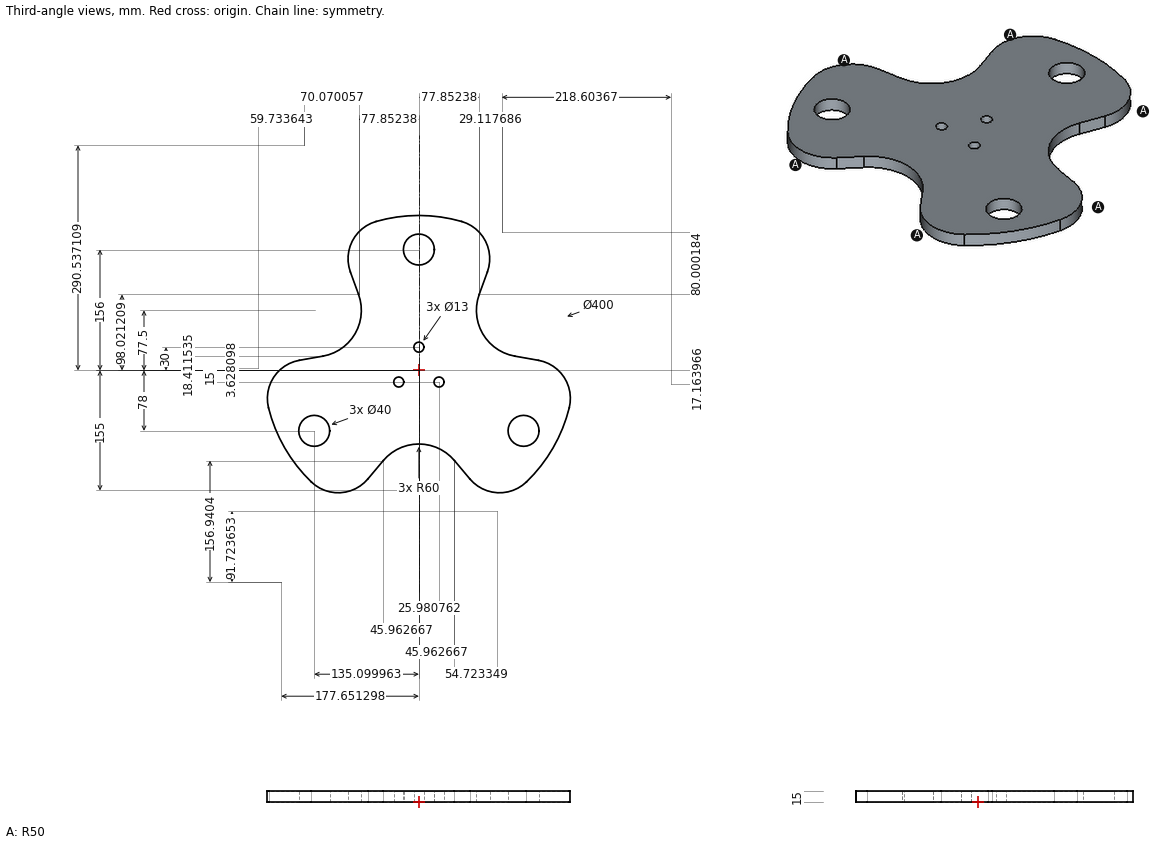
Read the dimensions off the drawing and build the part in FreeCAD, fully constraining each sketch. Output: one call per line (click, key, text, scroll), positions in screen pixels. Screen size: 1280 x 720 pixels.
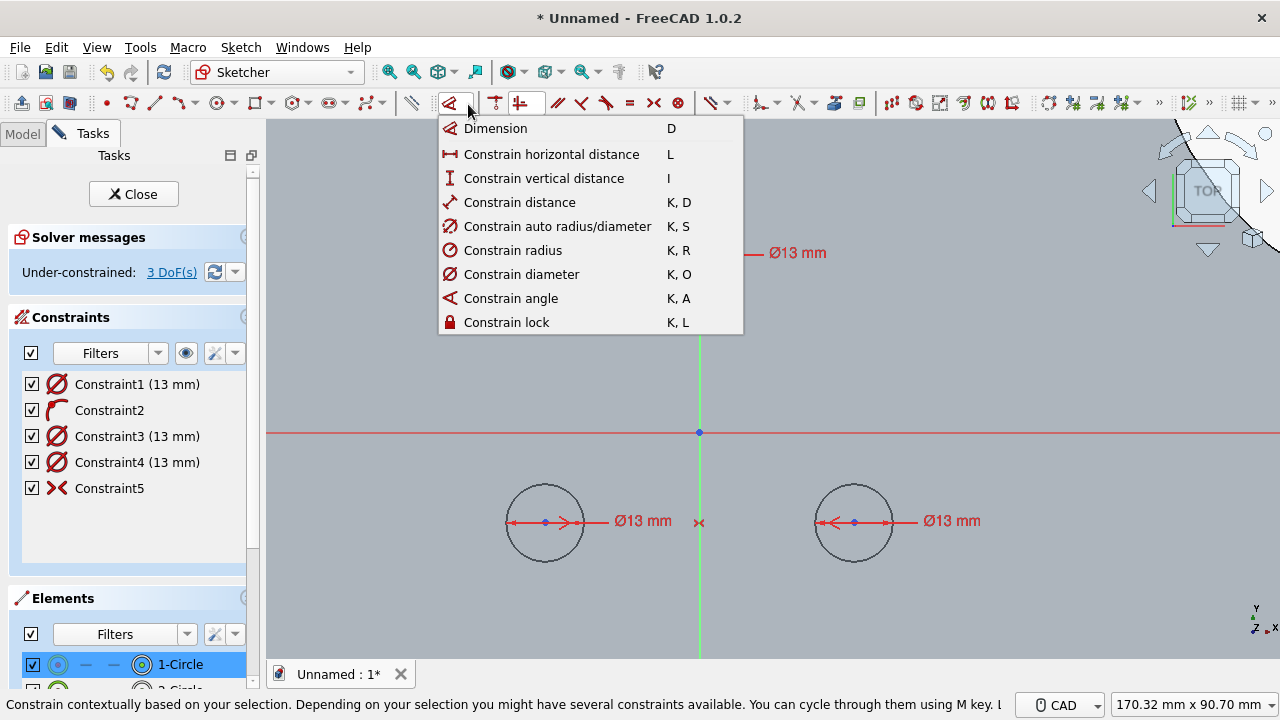
click(591, 178)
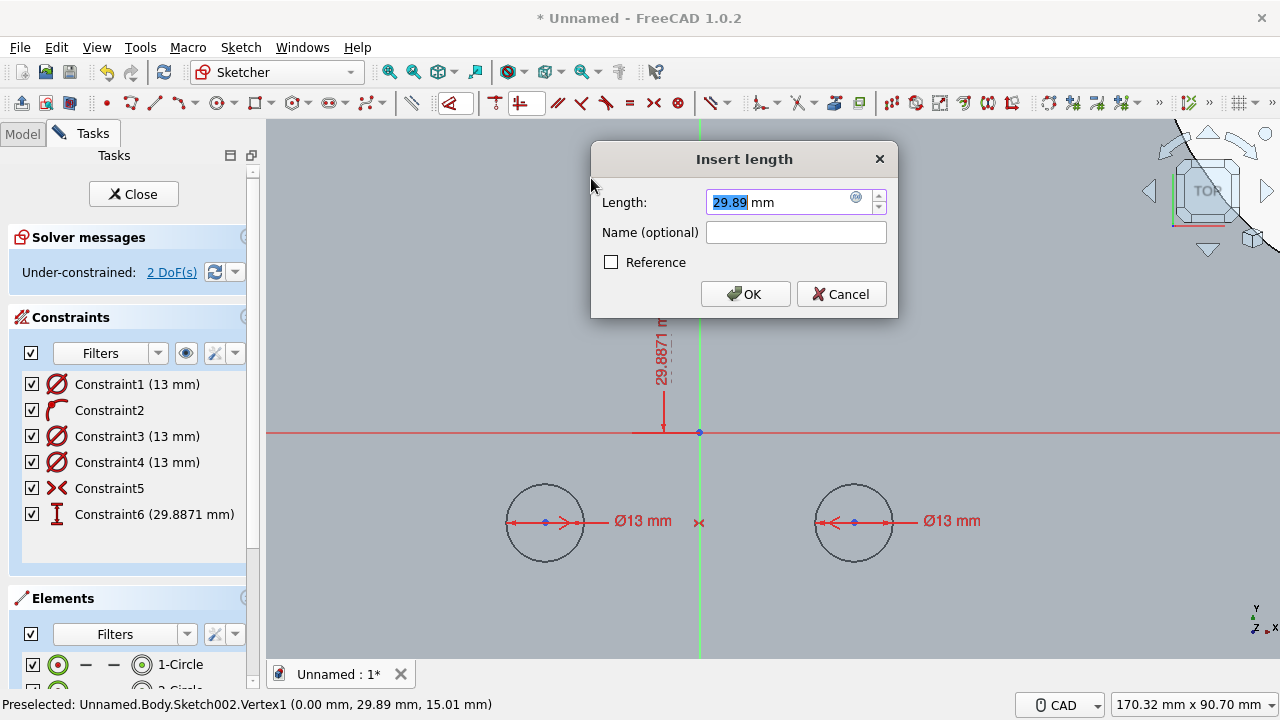
text(30)
key(Return)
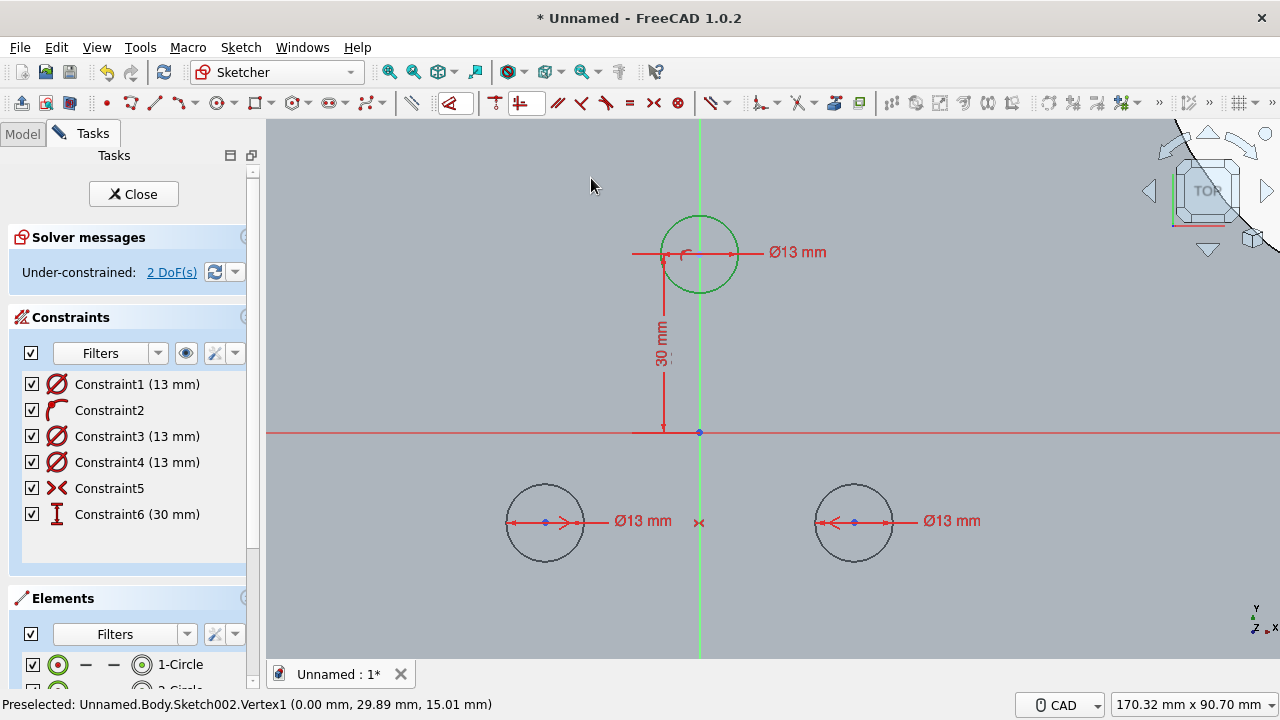
click(854, 523)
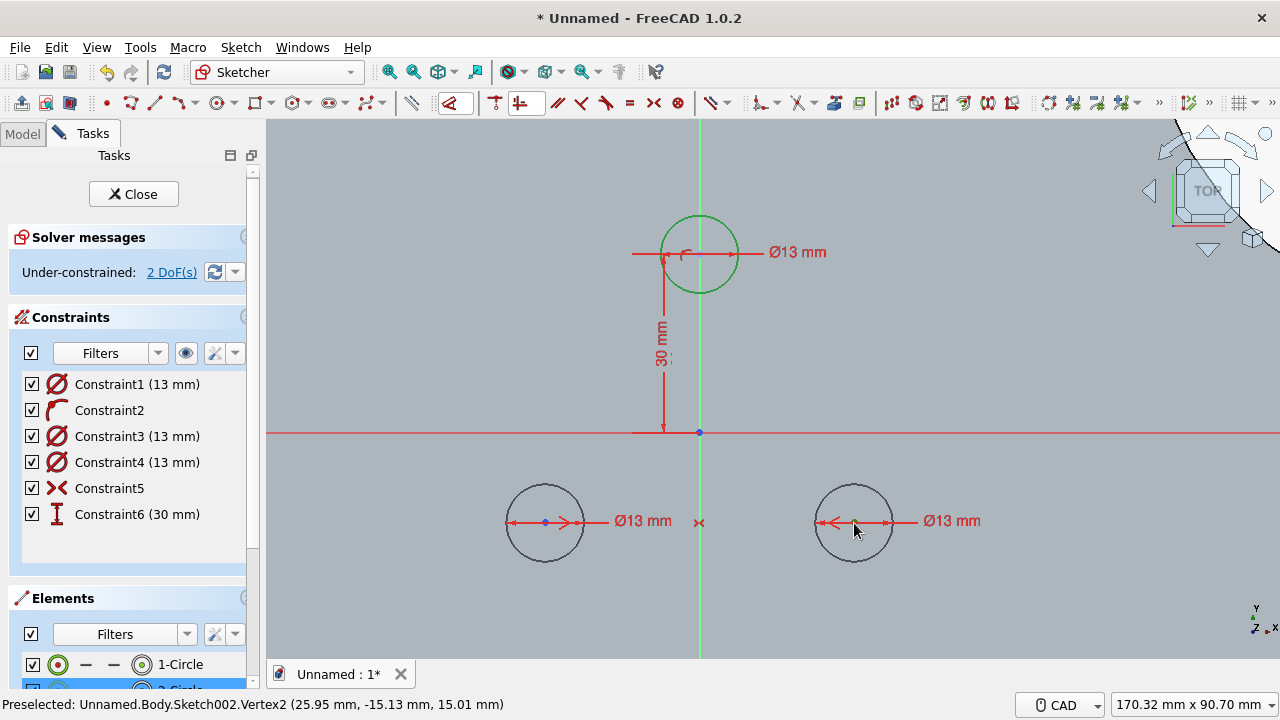
key(i)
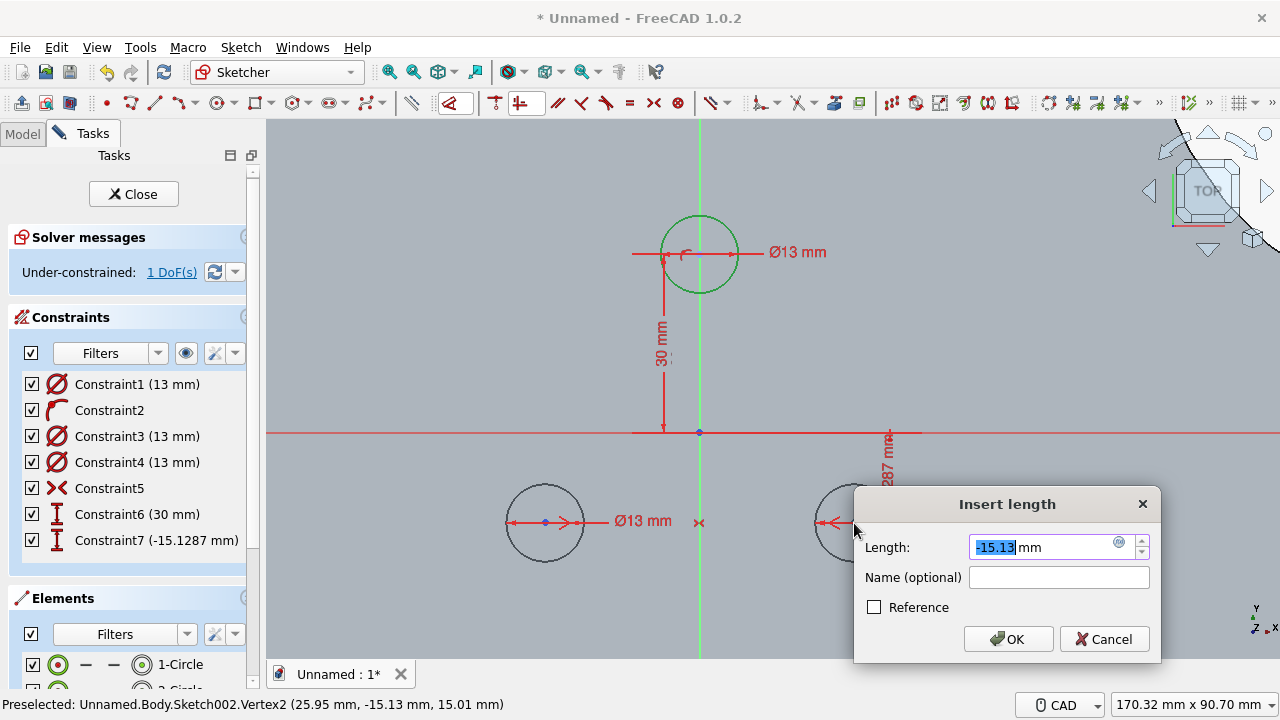
text(-15)
key(Return)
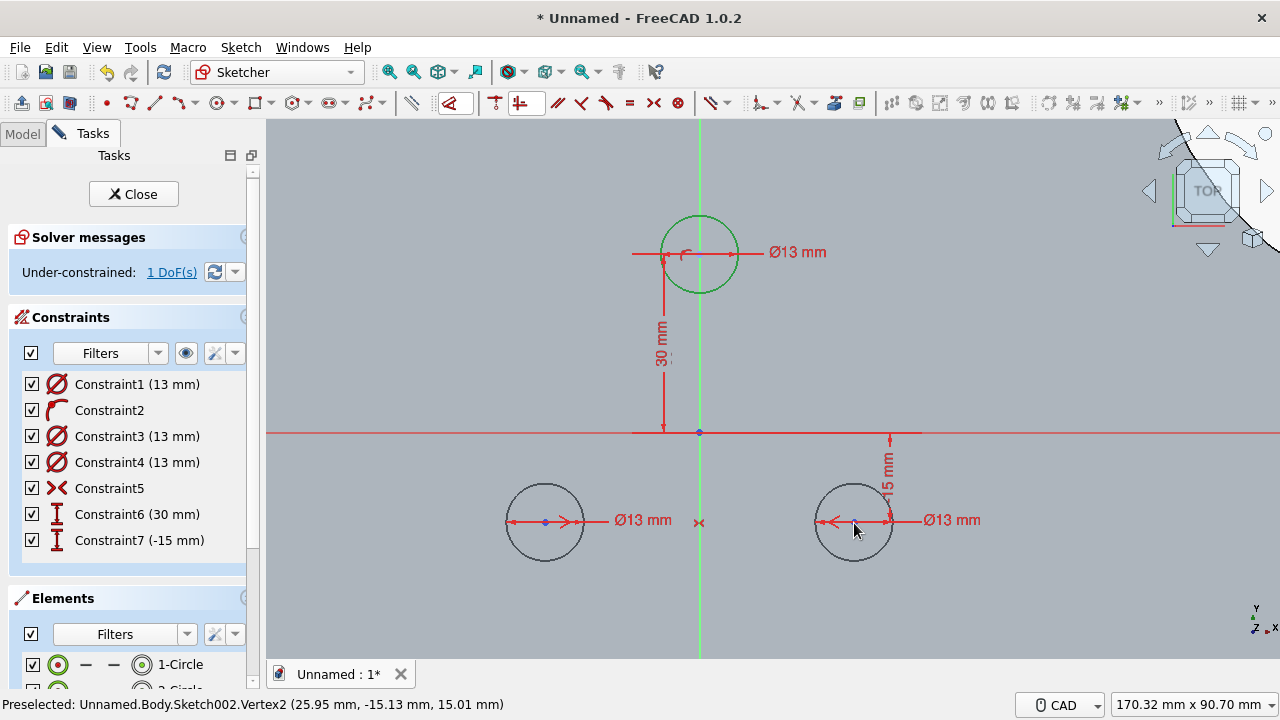
click(854, 522)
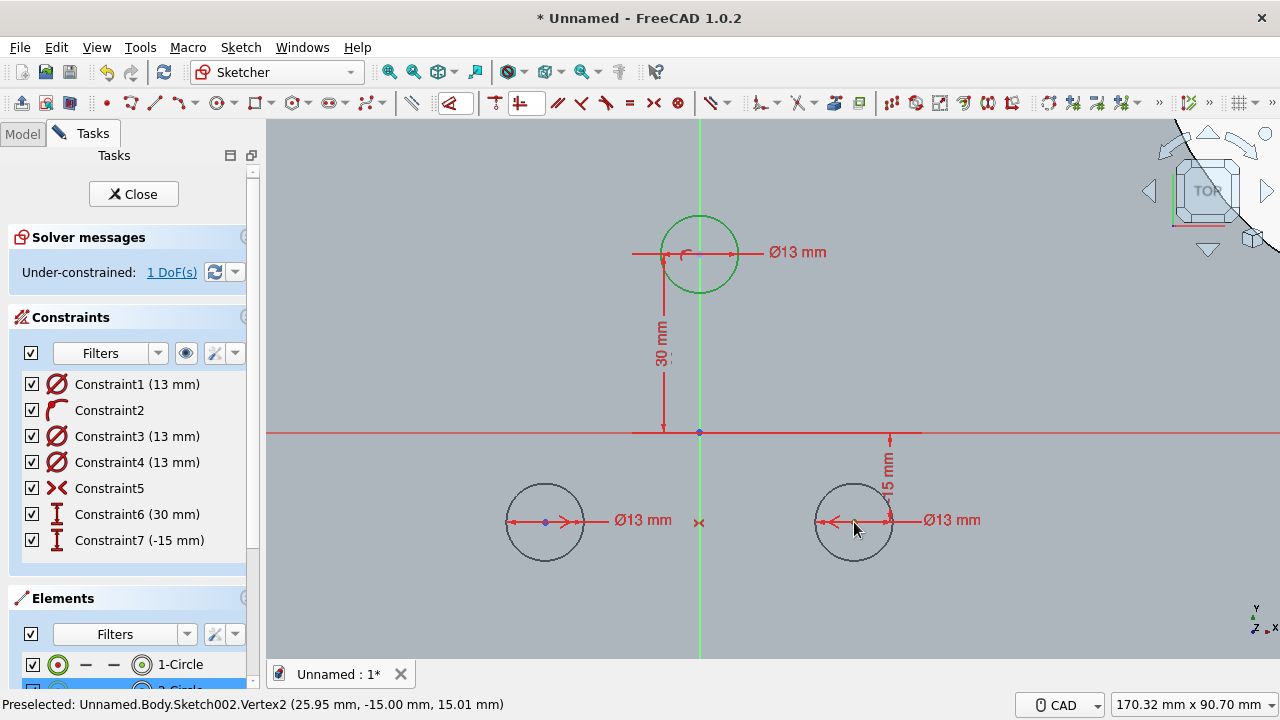
click(468, 104)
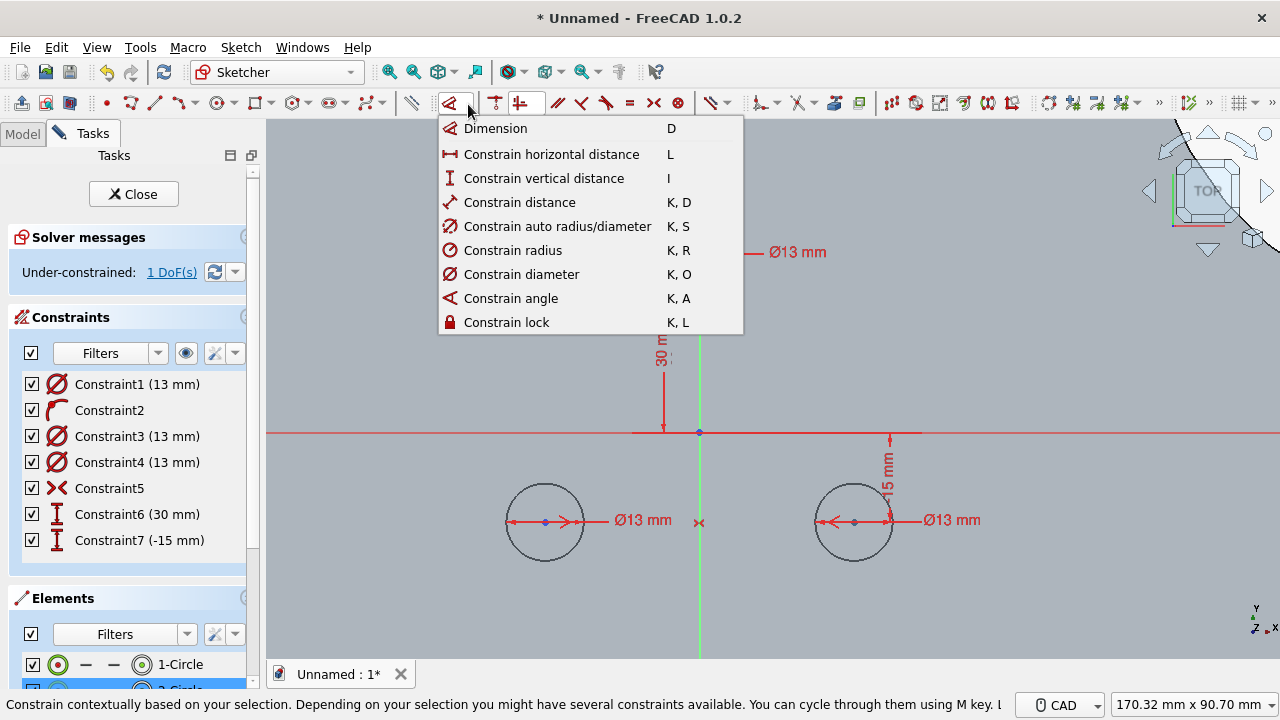
click(591, 154)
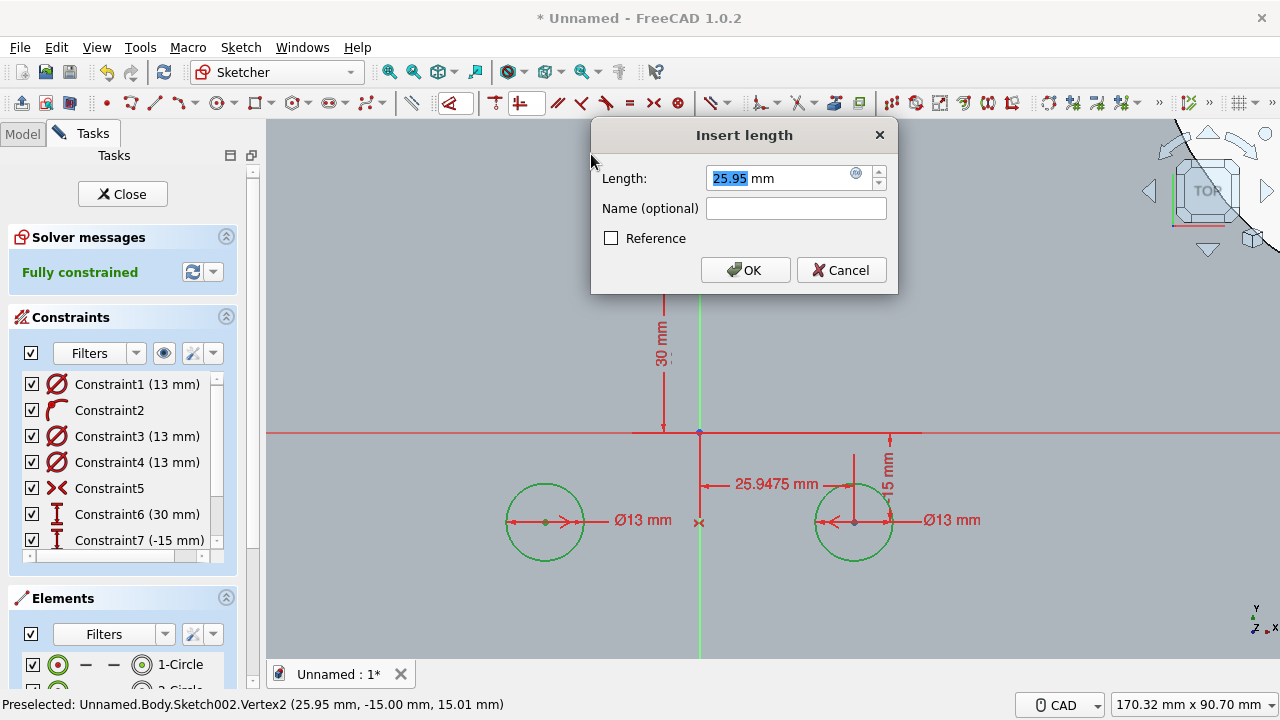
text(25.980762)
key(Return)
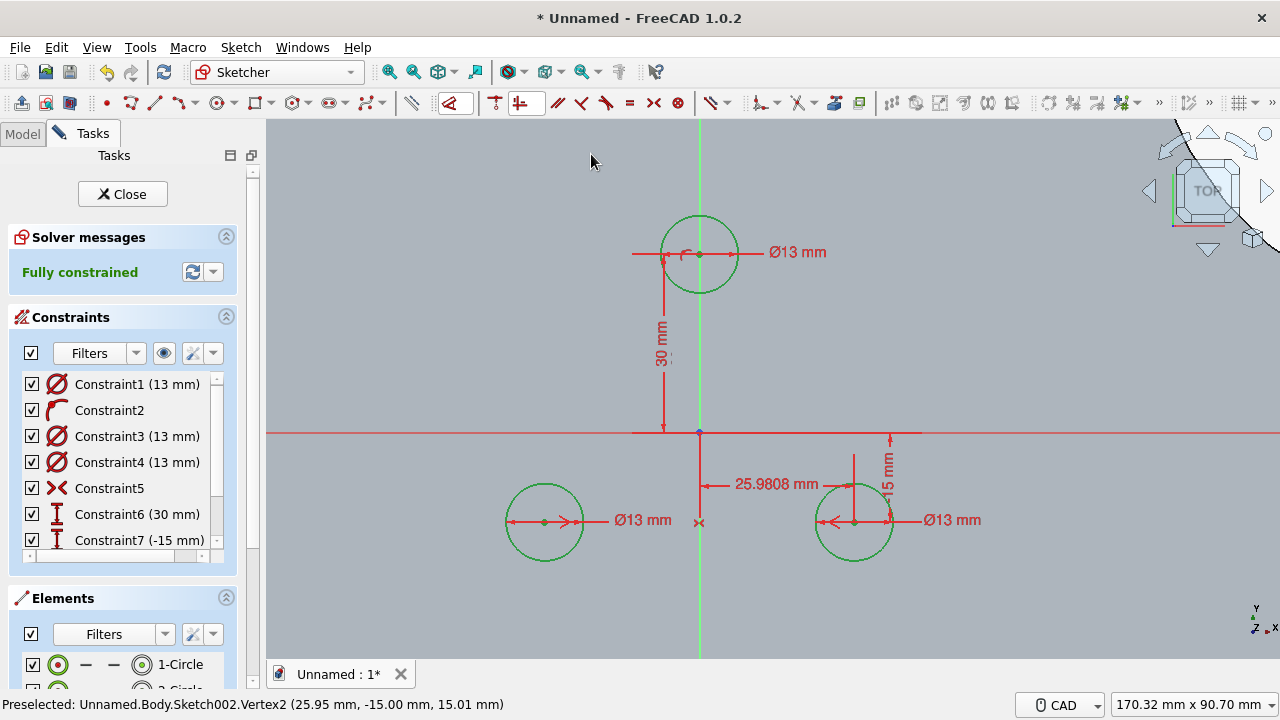
click(123, 194)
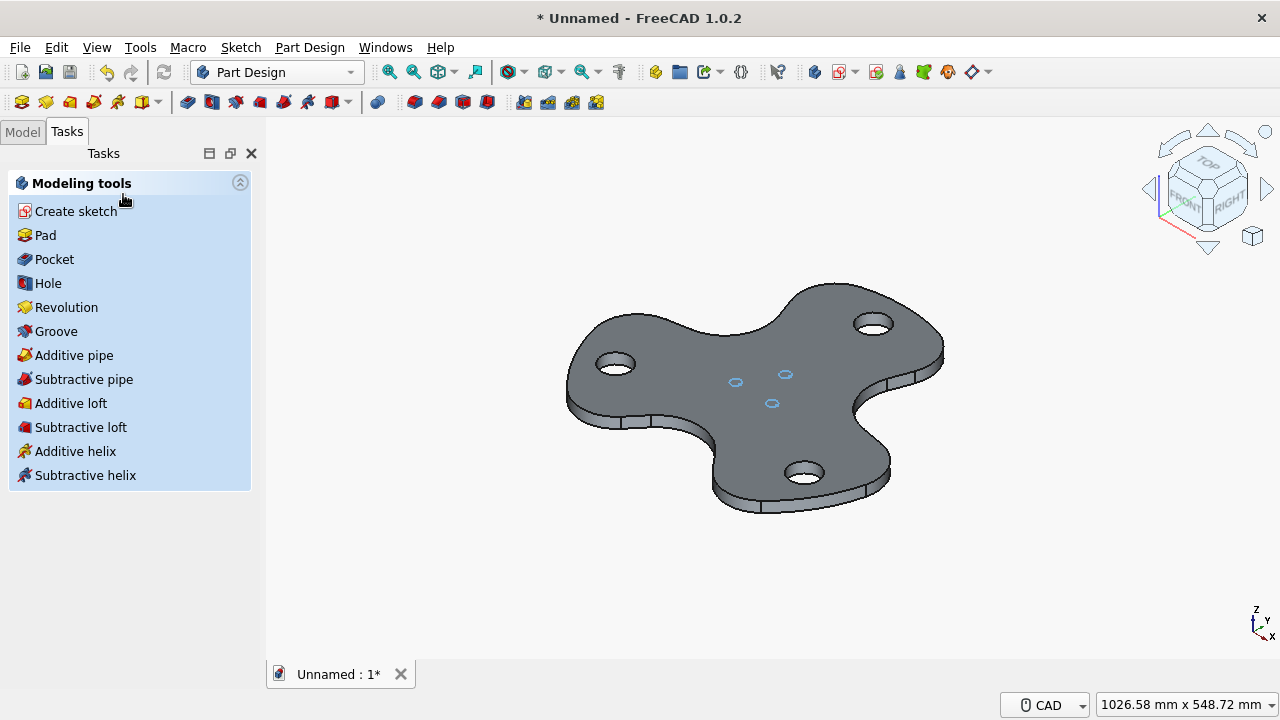
click(188, 102)